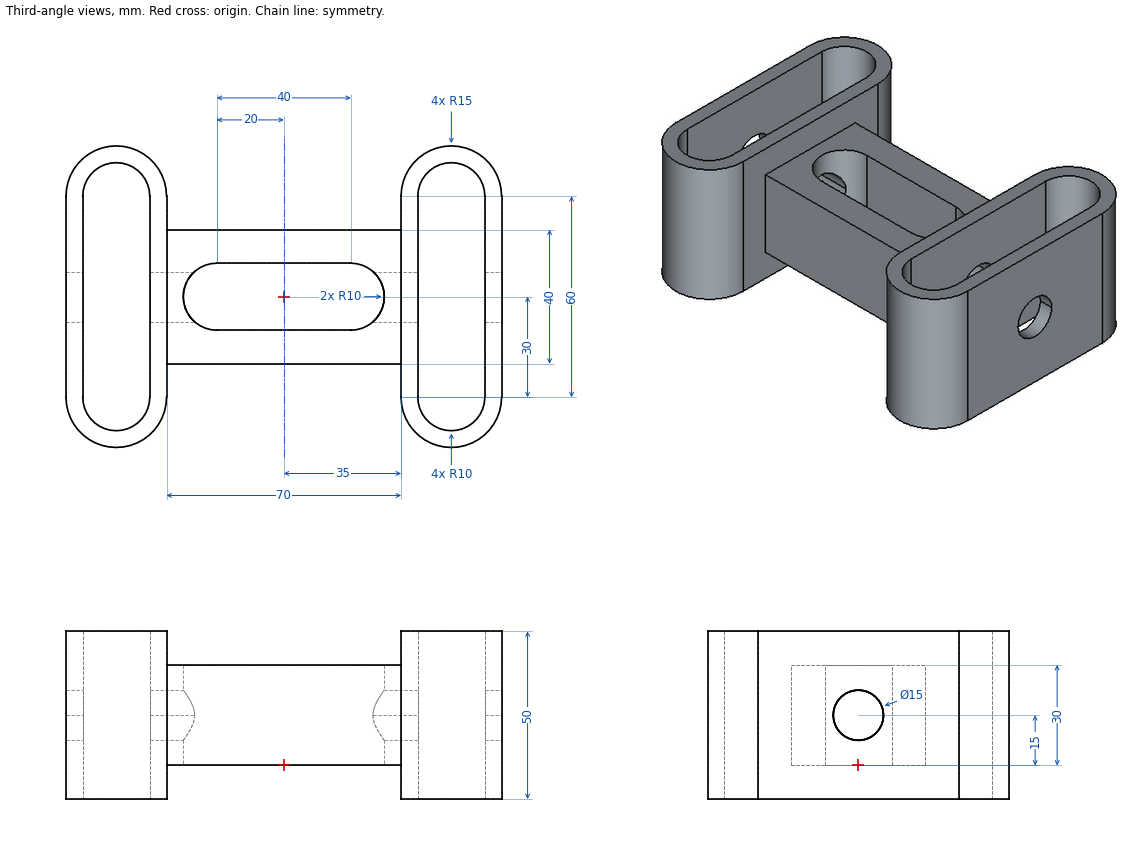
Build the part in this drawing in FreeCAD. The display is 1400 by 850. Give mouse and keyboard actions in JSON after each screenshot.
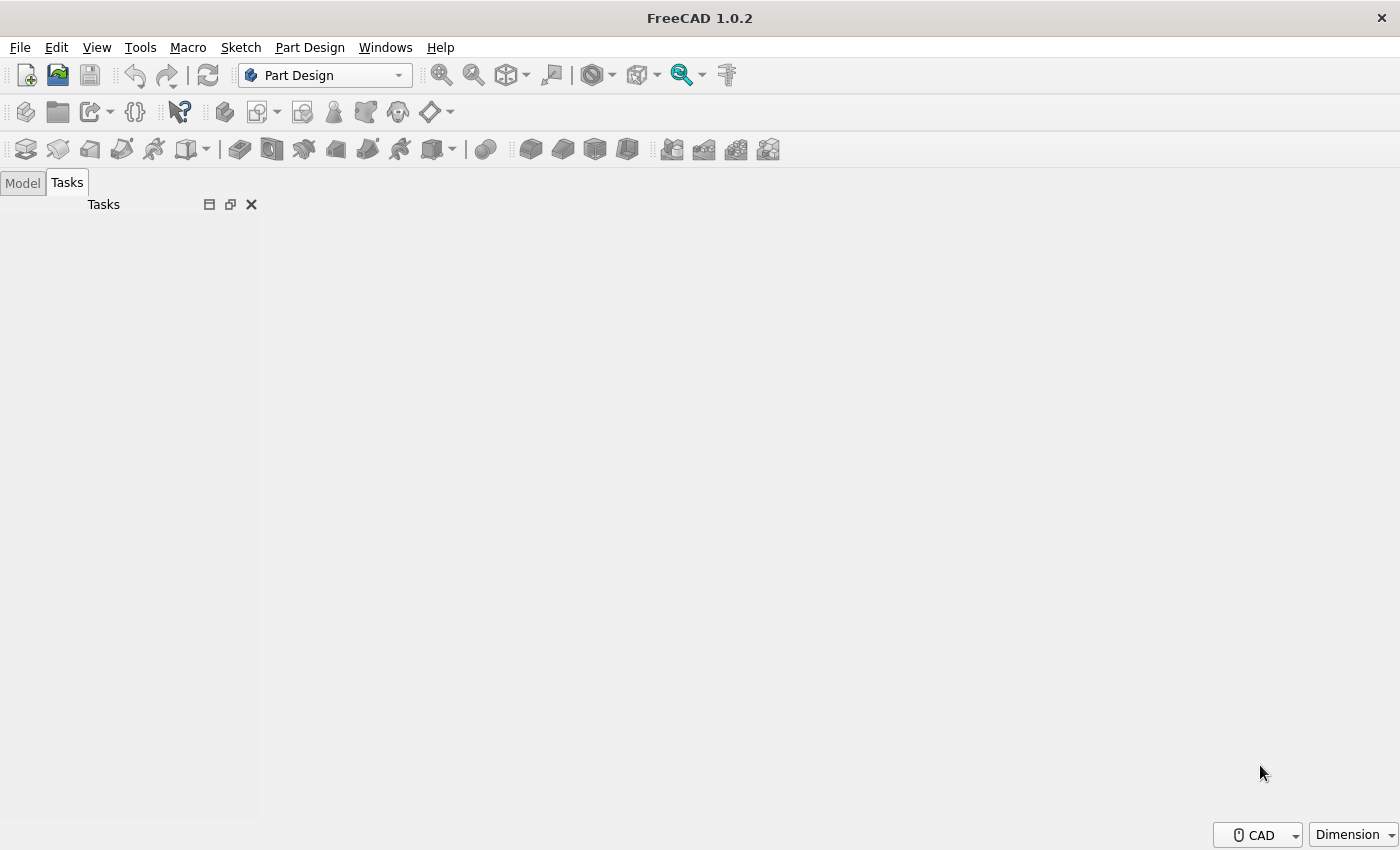
{"action": "key", "text": "ctrl+n"}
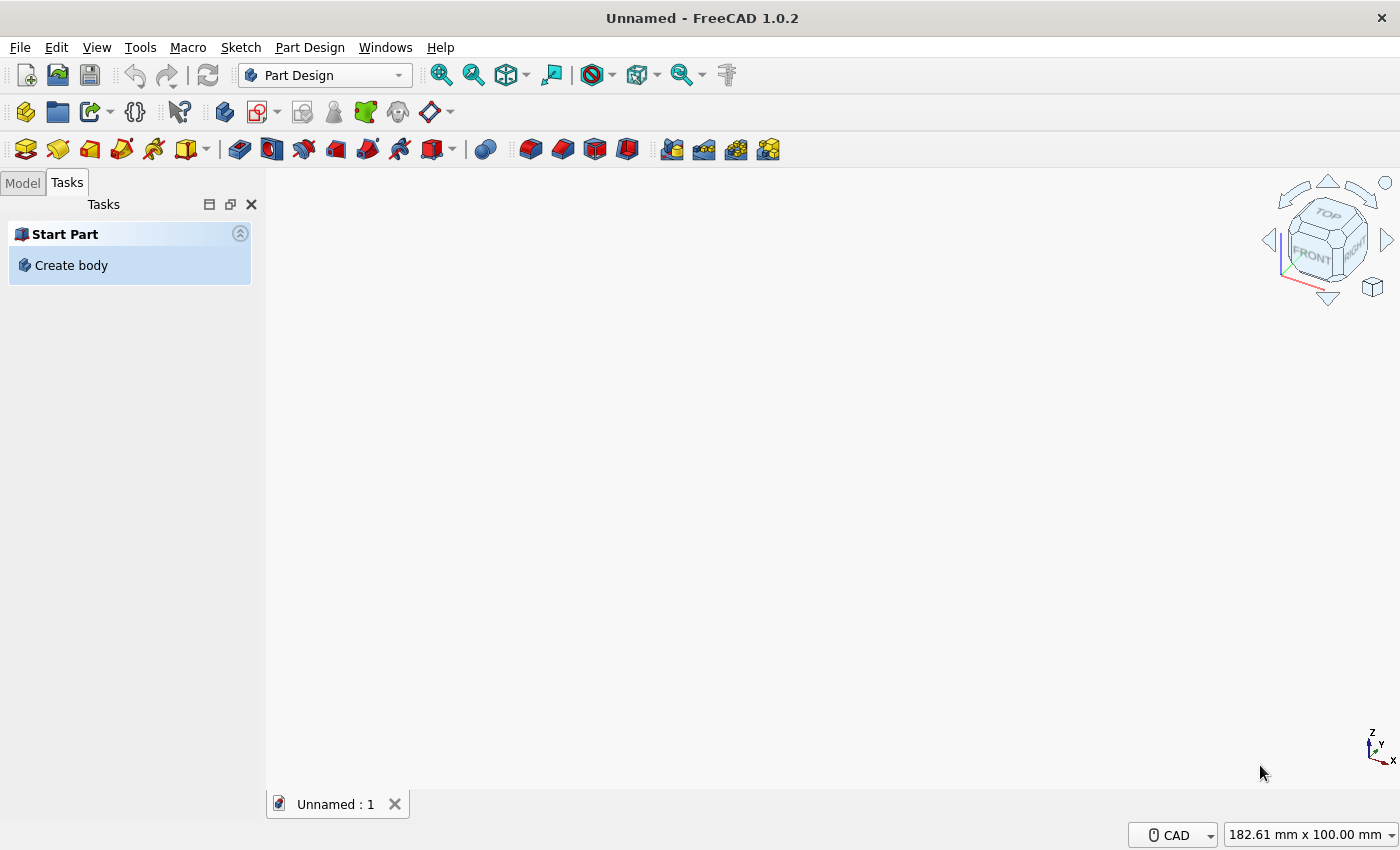
{"action": "left_click", "coordinate": [258, 112]}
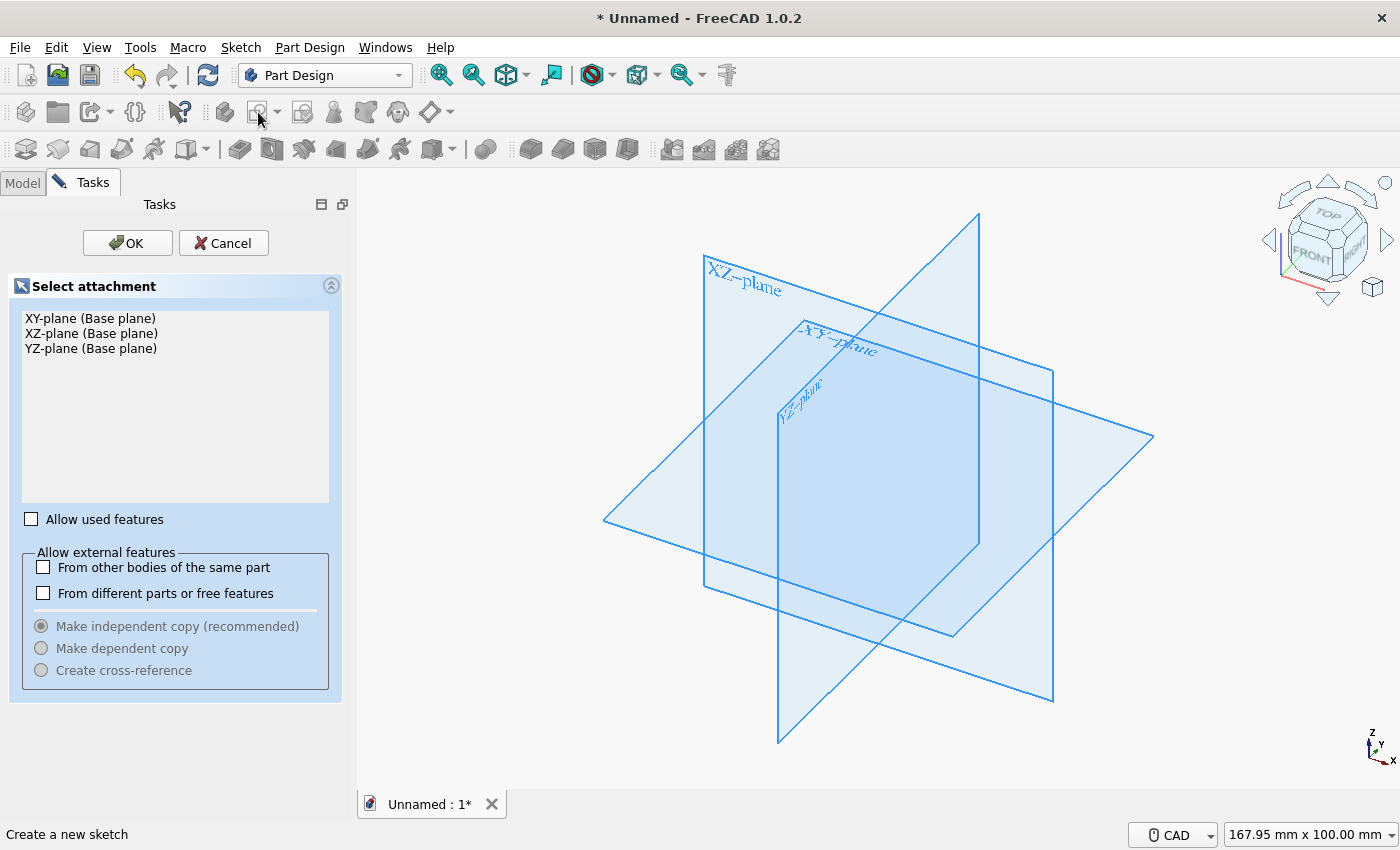
{"action": "left_click", "coordinate": [82, 318]}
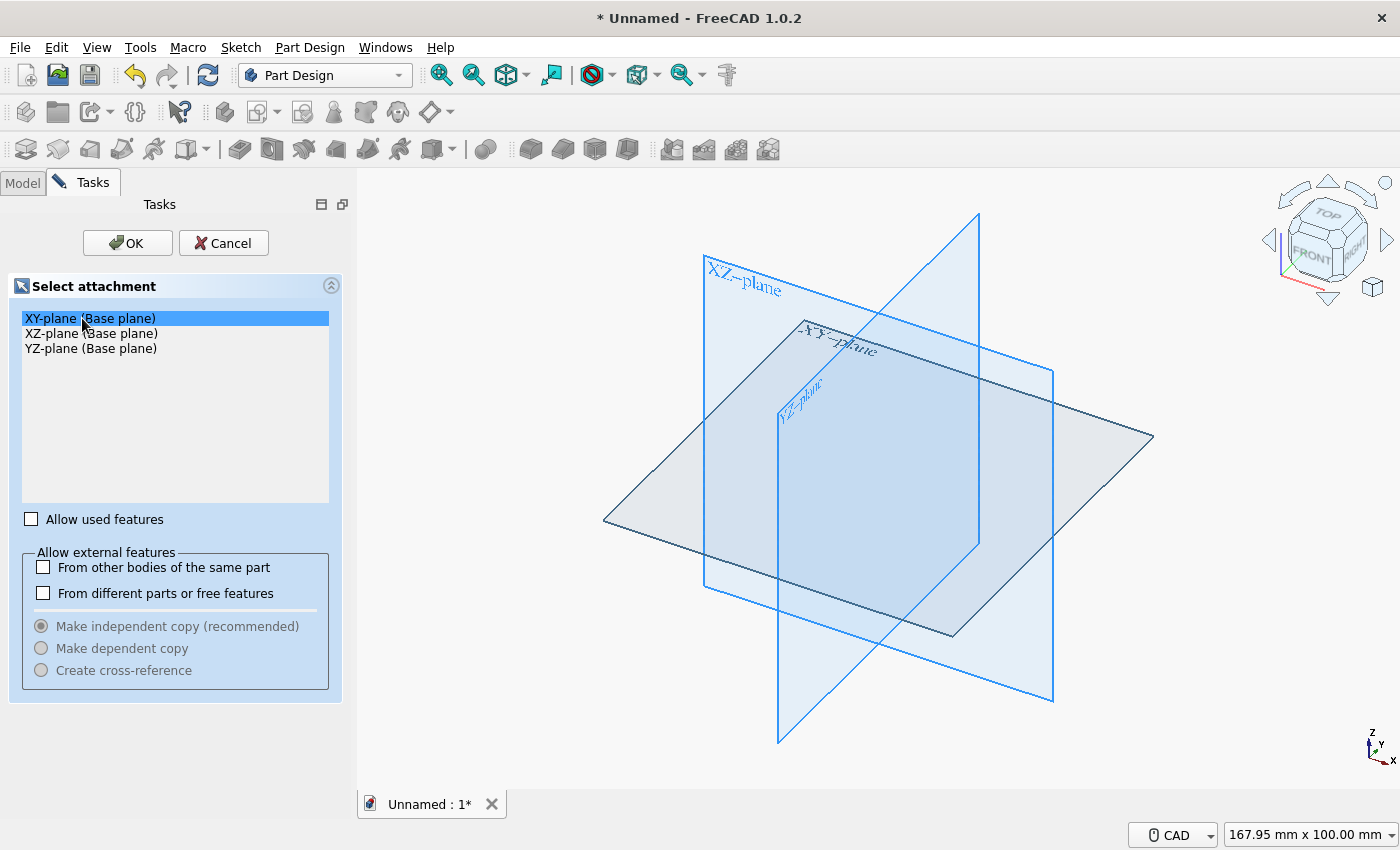
{"action": "left_click", "coordinate": [128, 243]}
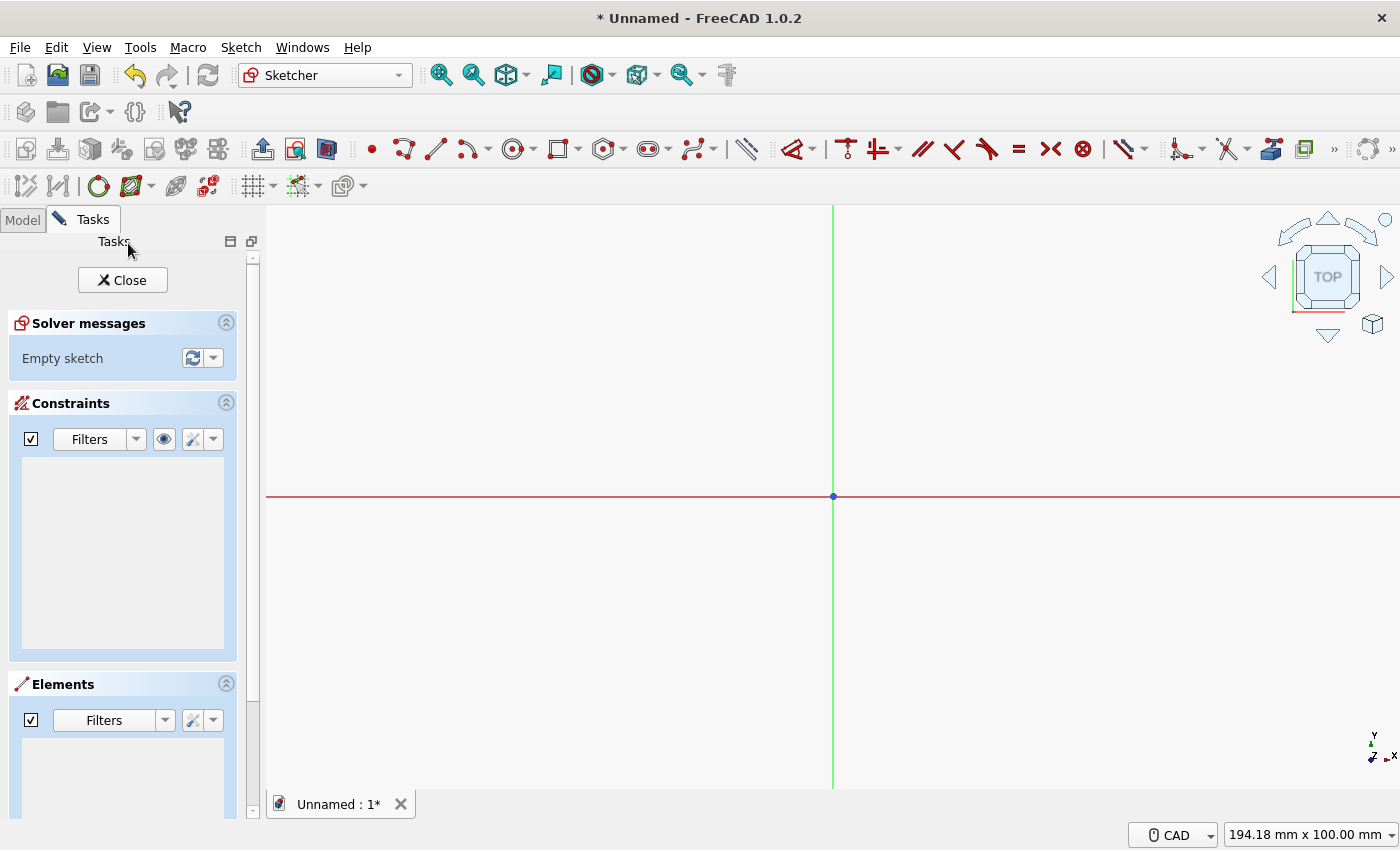
{"action": "scroll", "coordinate": [972, 497], "scroll_direction": "up", "scroll_amount": 2}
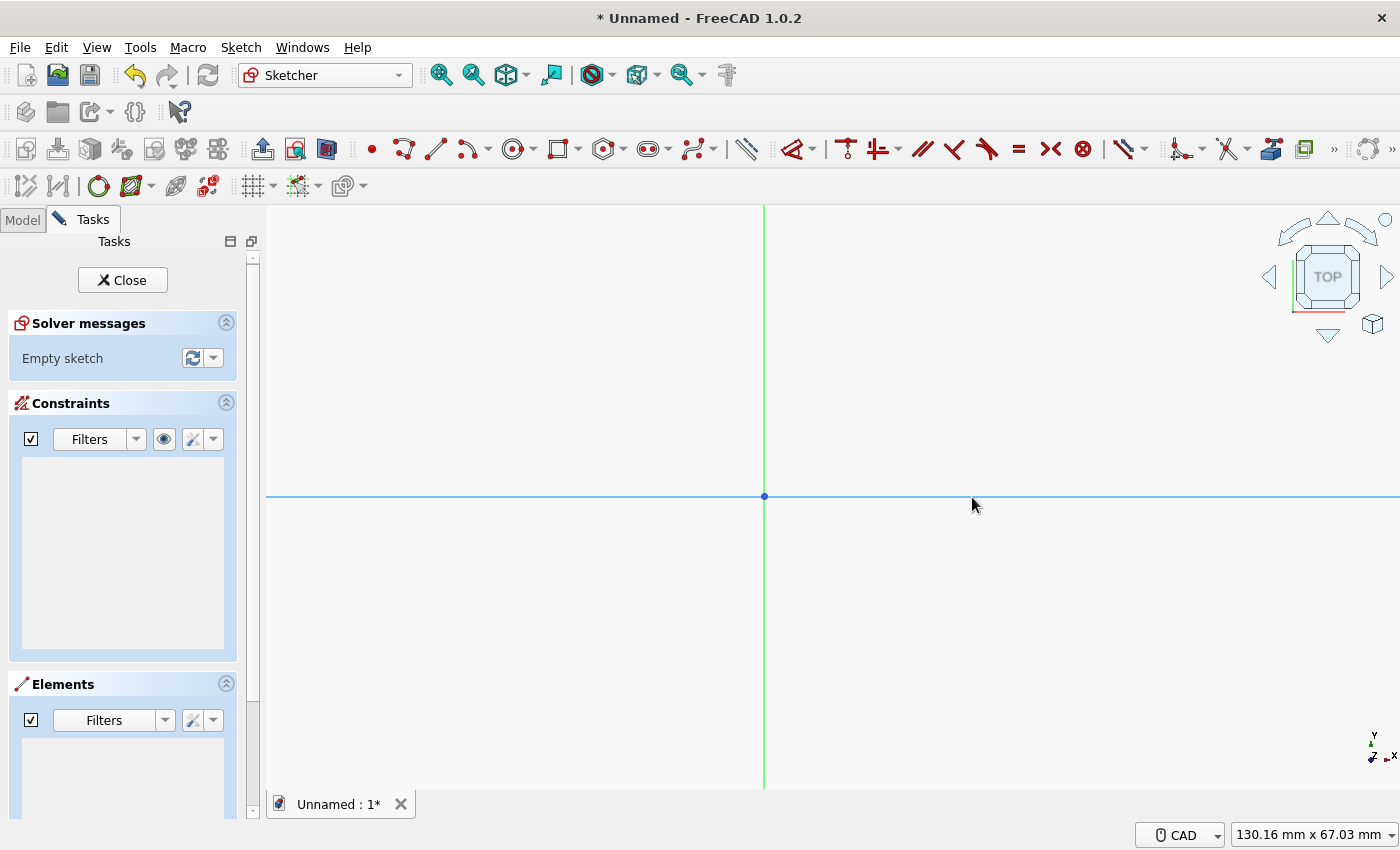
{"action": "key", "text": "g v"}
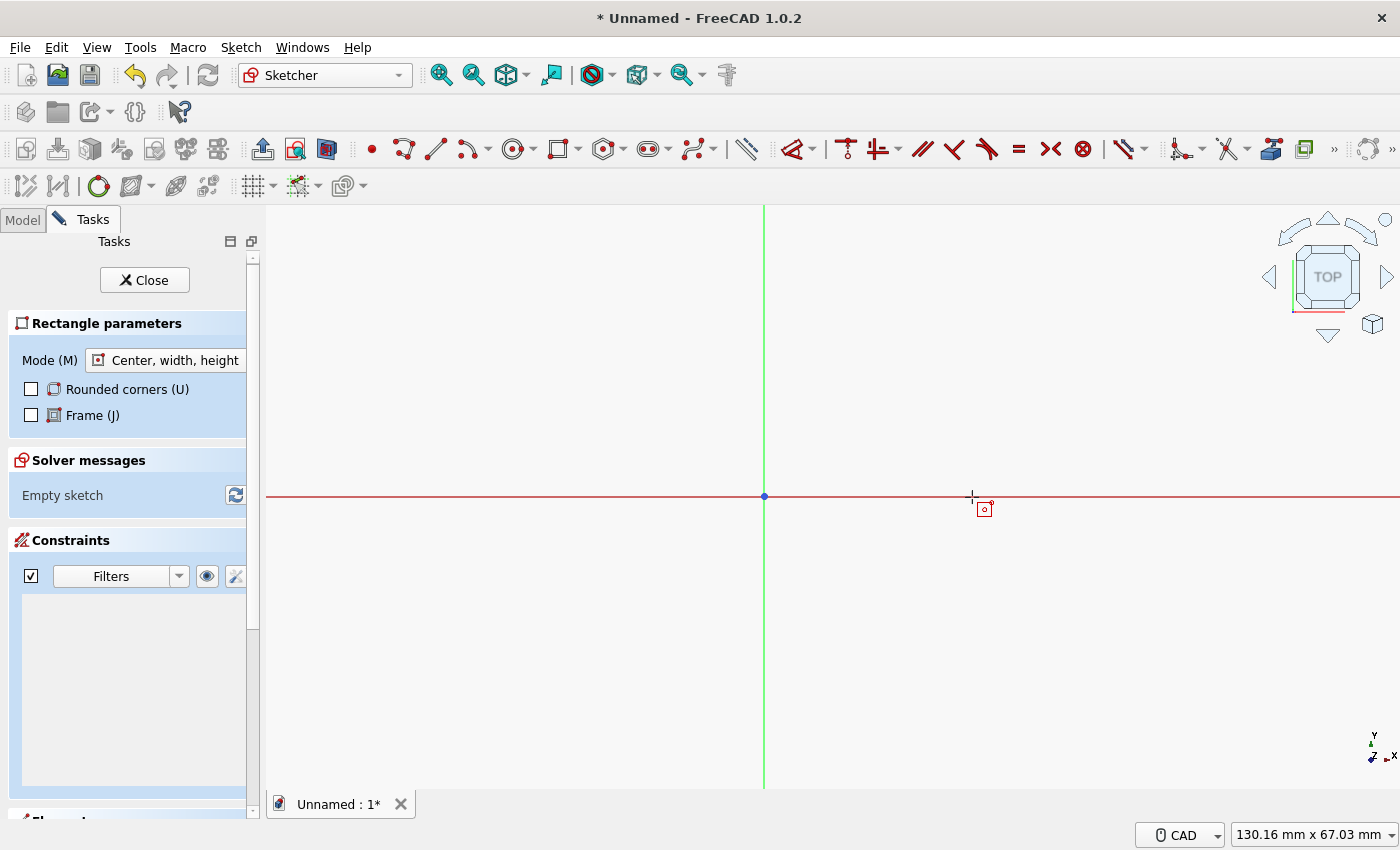
{"action": "left_click", "coordinate": [764, 497]}
{"action": "mouse_move", "coordinate": [1069, 323]}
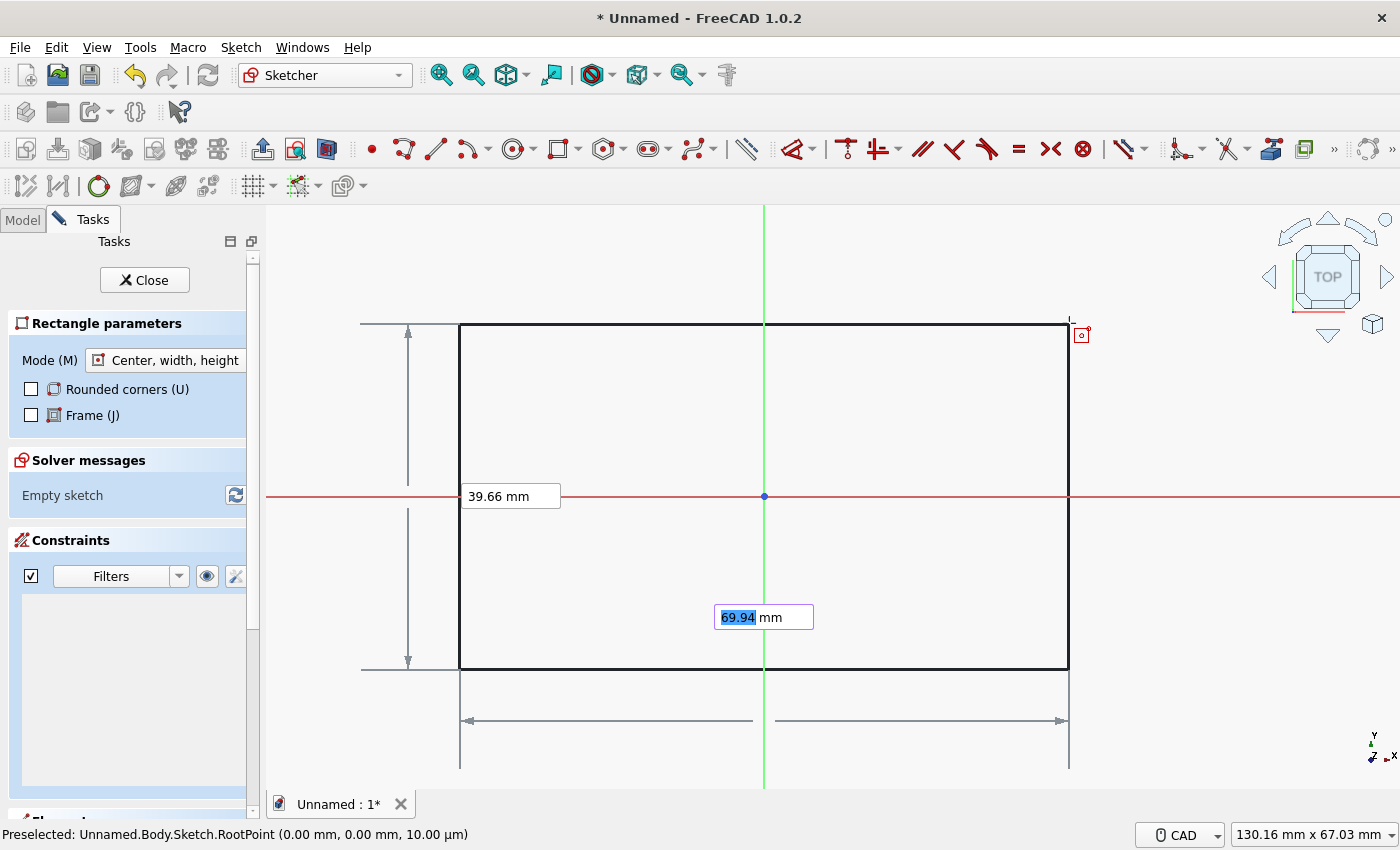
{"action": "type", "text": "70"}
{"action": "key", "text": "Tab"}
{"action": "type", "text": "40"}
{"action": "key", "text": "Return"}